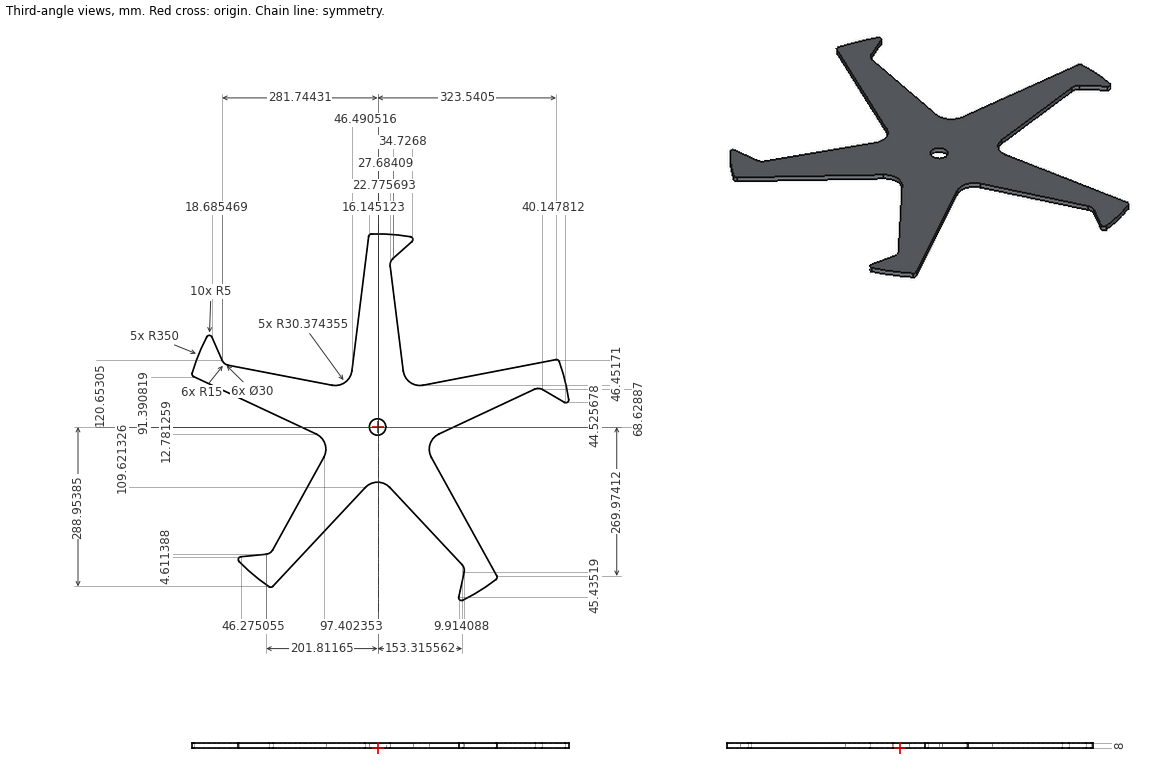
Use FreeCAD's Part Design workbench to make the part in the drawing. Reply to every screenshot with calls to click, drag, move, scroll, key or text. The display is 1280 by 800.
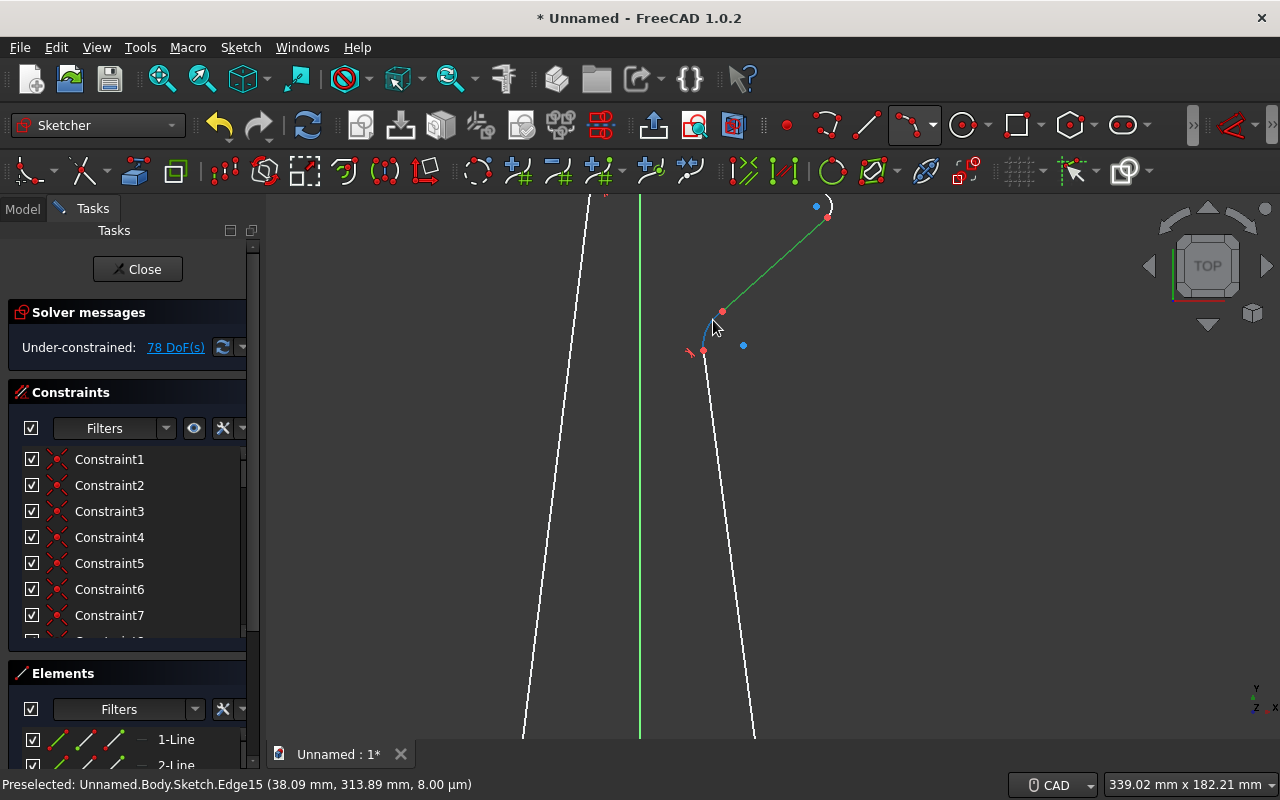
click(712, 320)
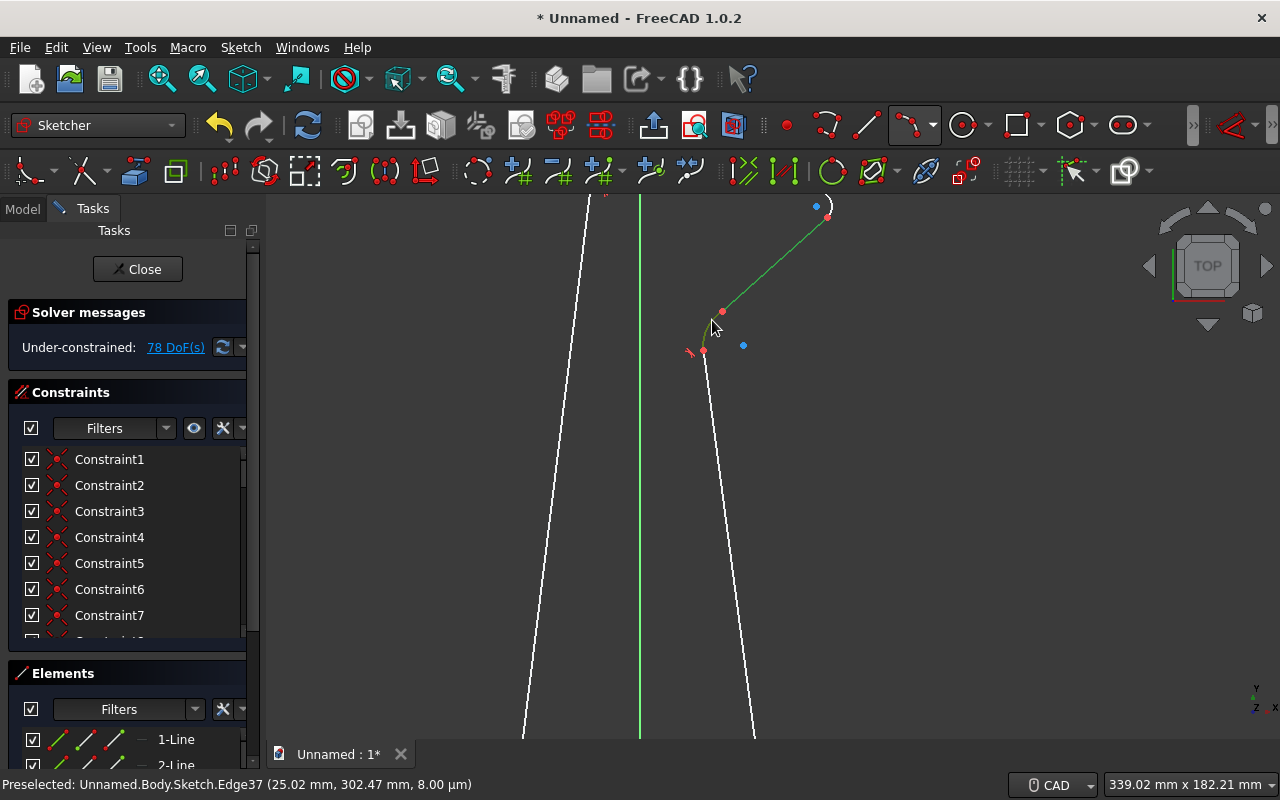
key(t)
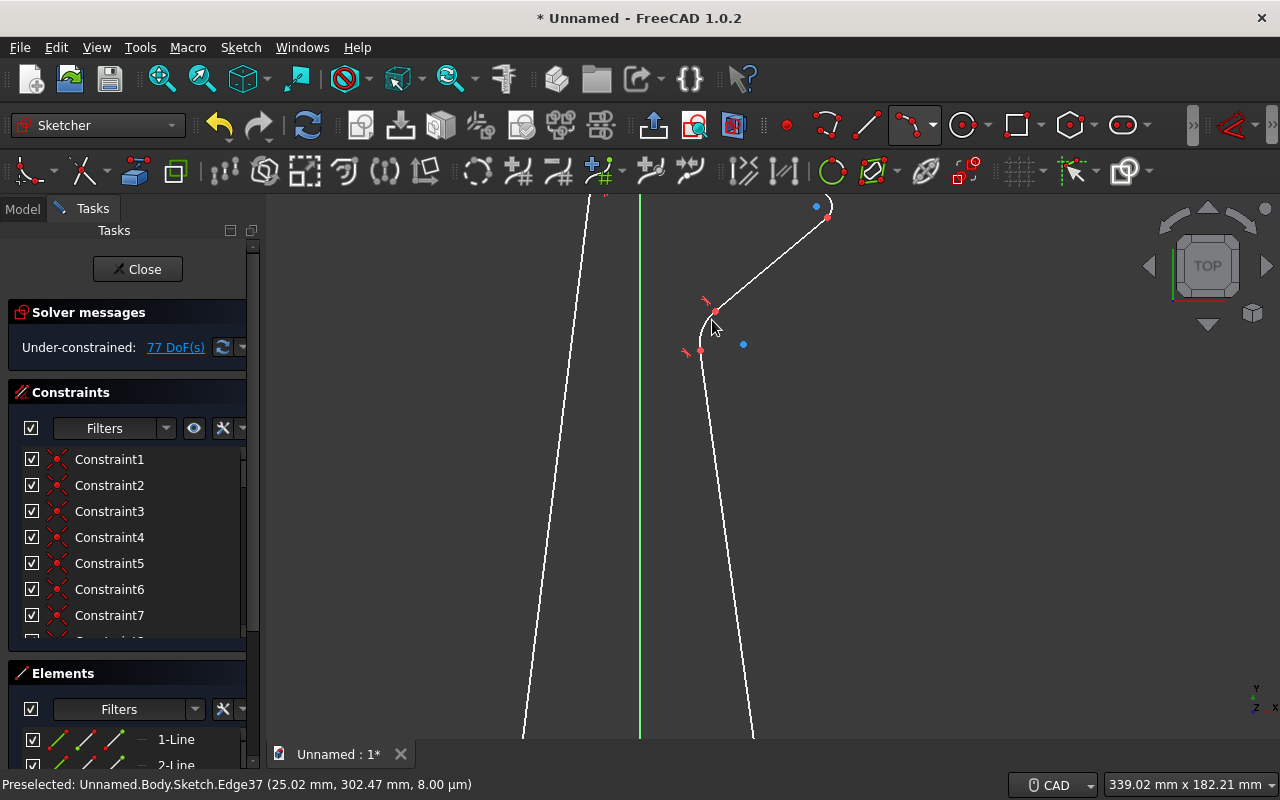
scroll(714, 327, down, 9)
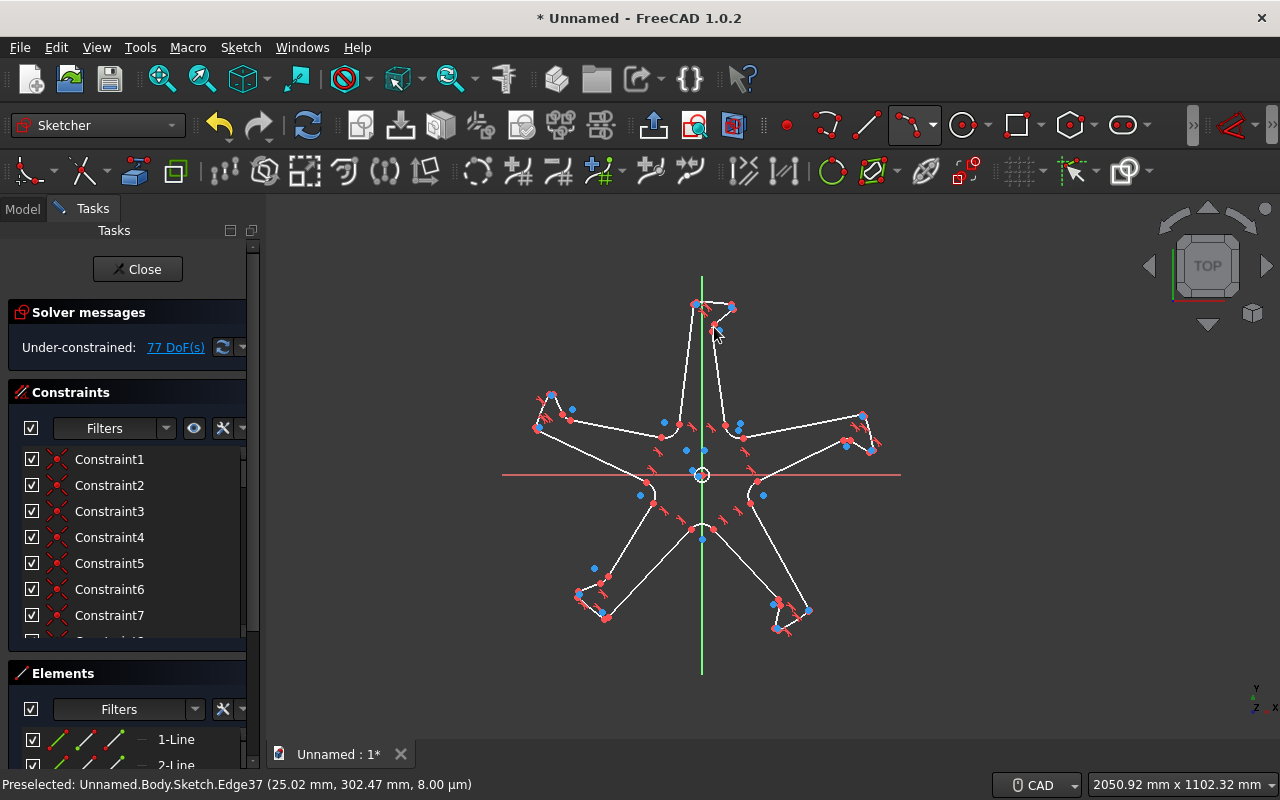
scroll(720, 320, up, 4)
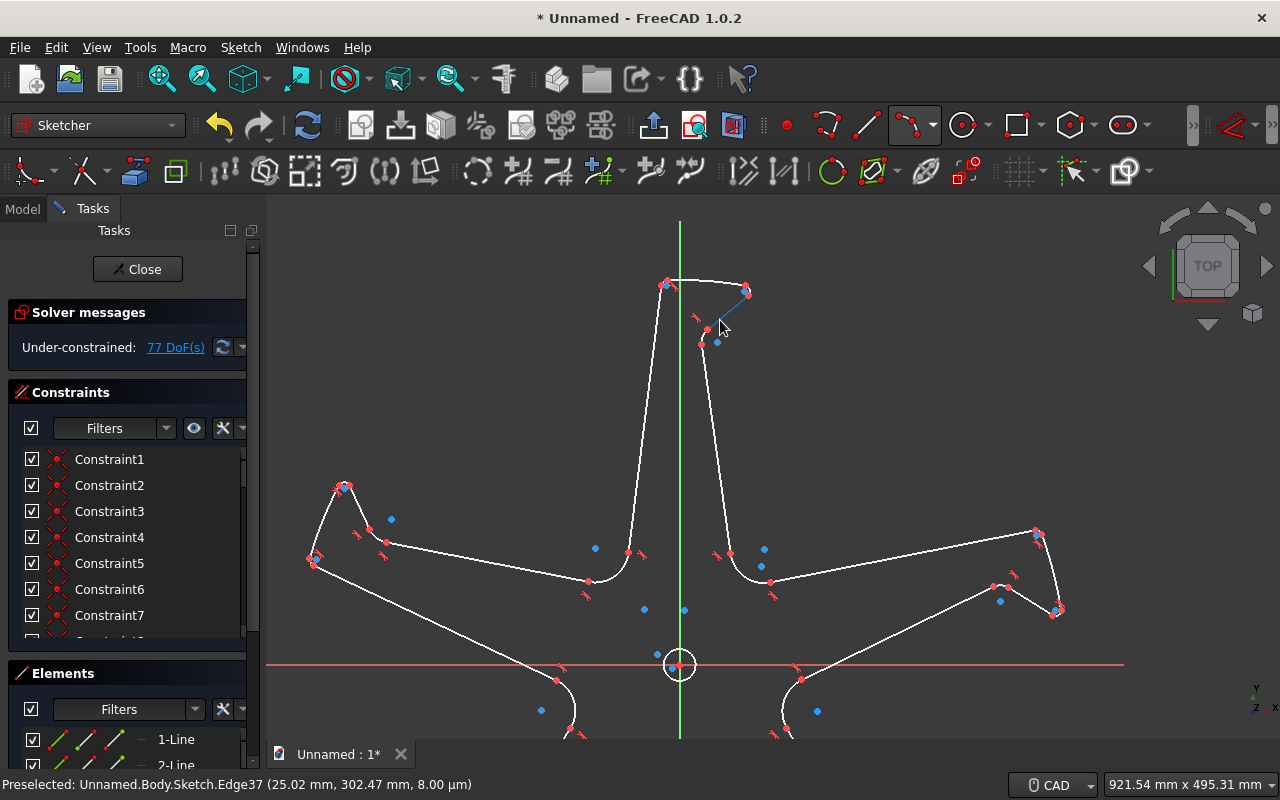
click(720, 320)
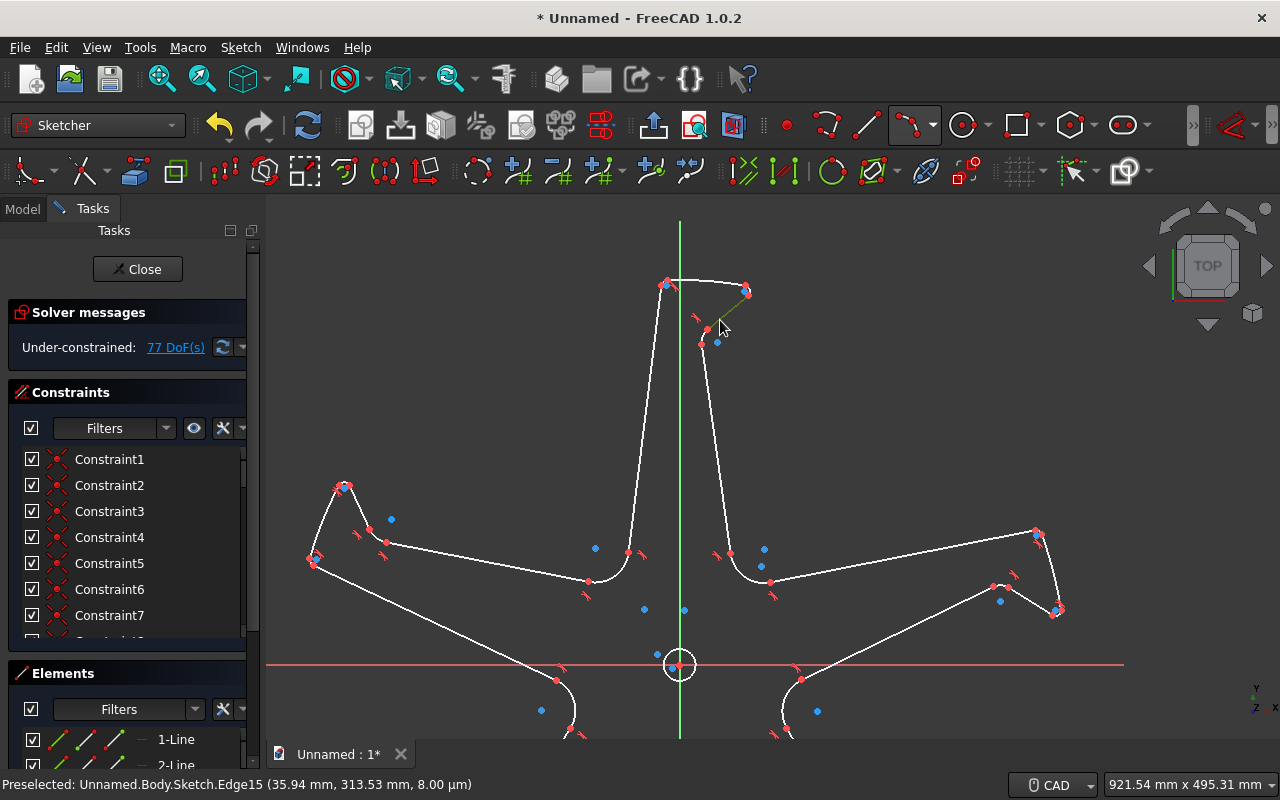
scroll(750, 290, up, 5)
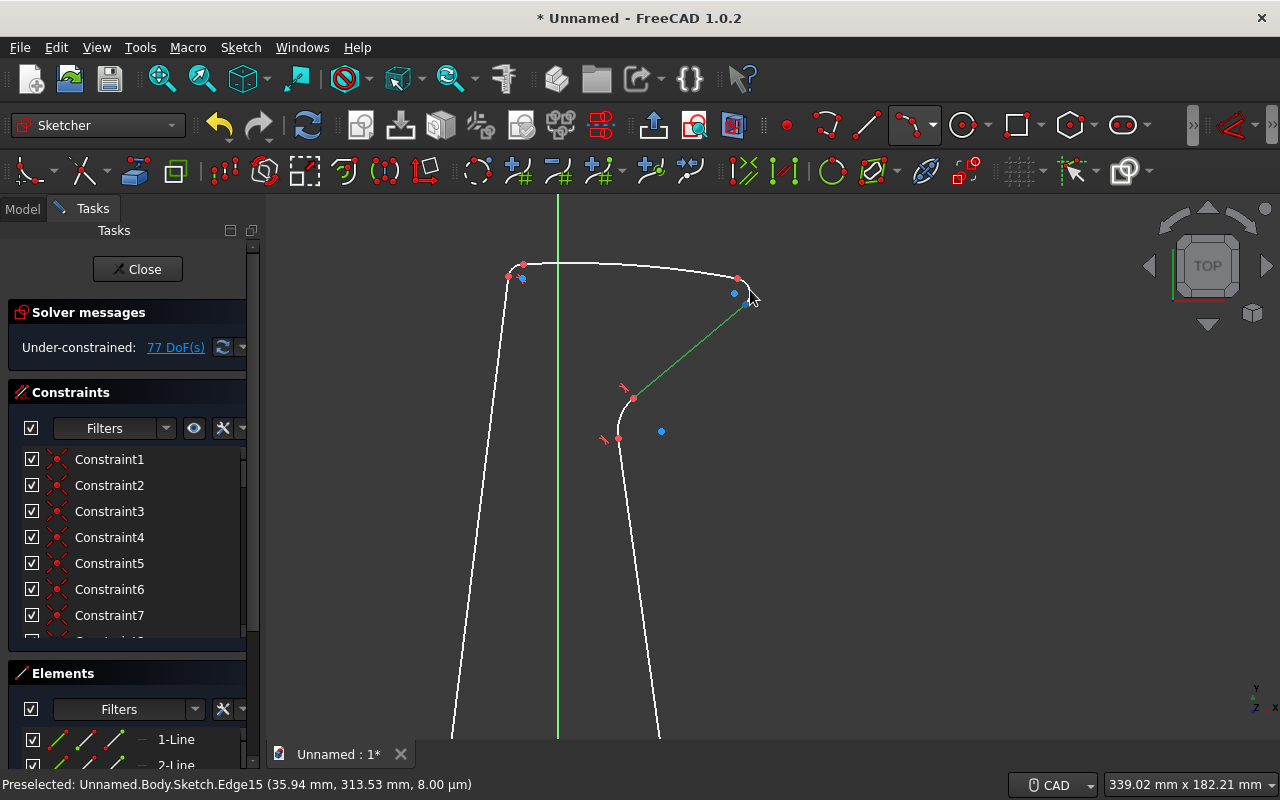
click(749, 289)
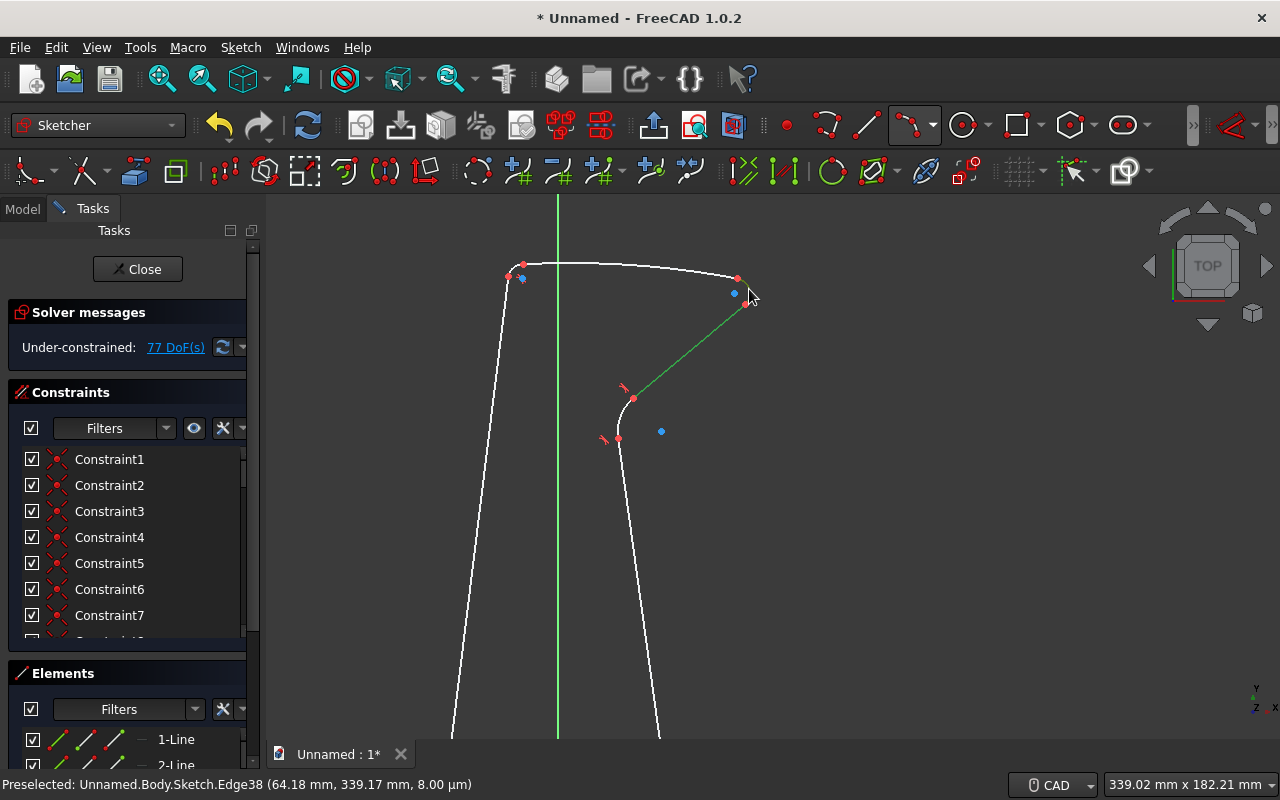
key(t)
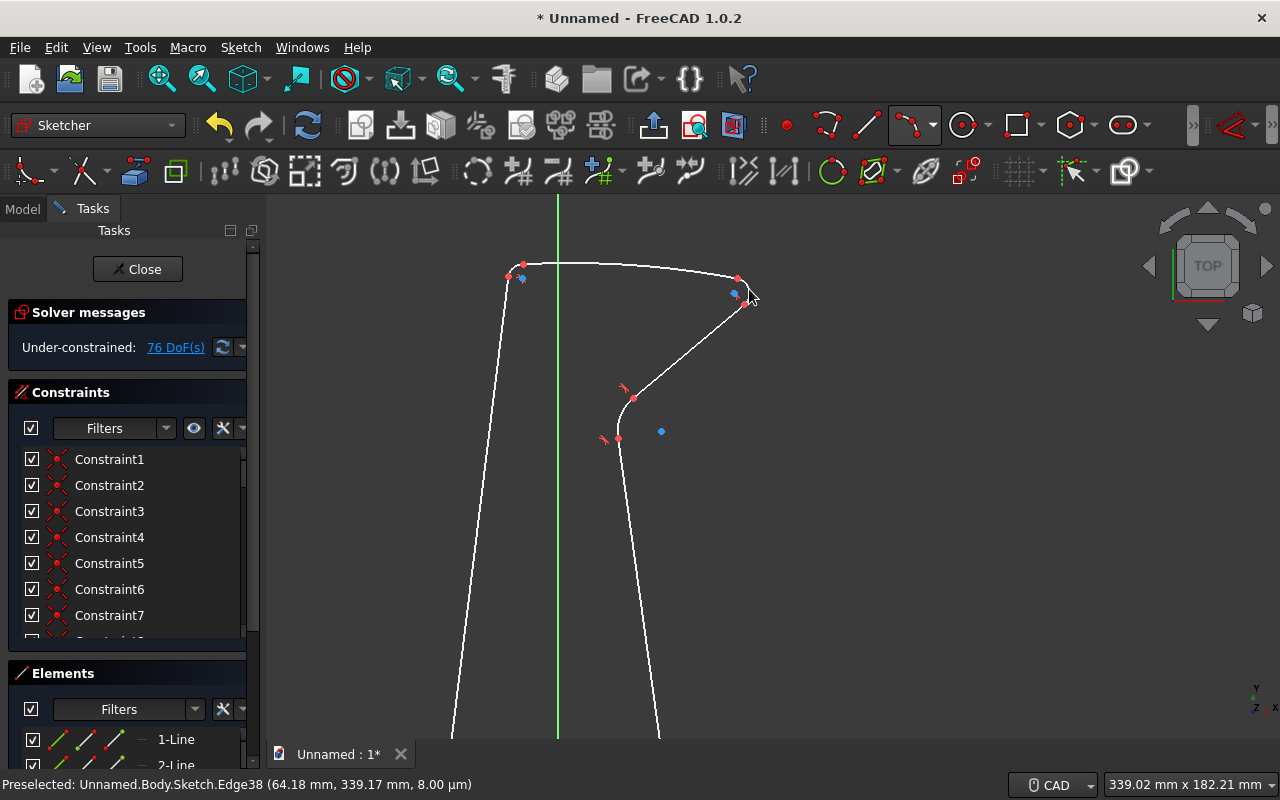
scroll(730, 310, down, 9)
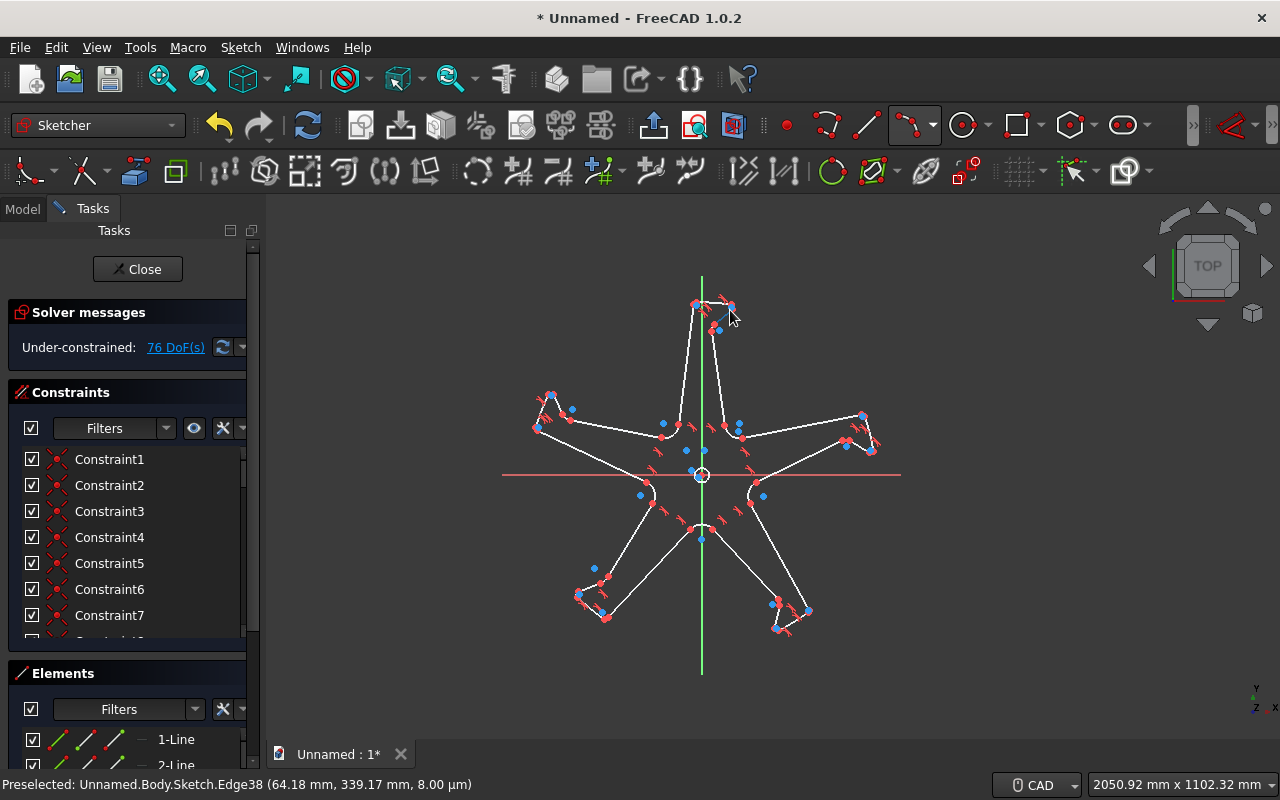
scroll(552, 394, up, 11)